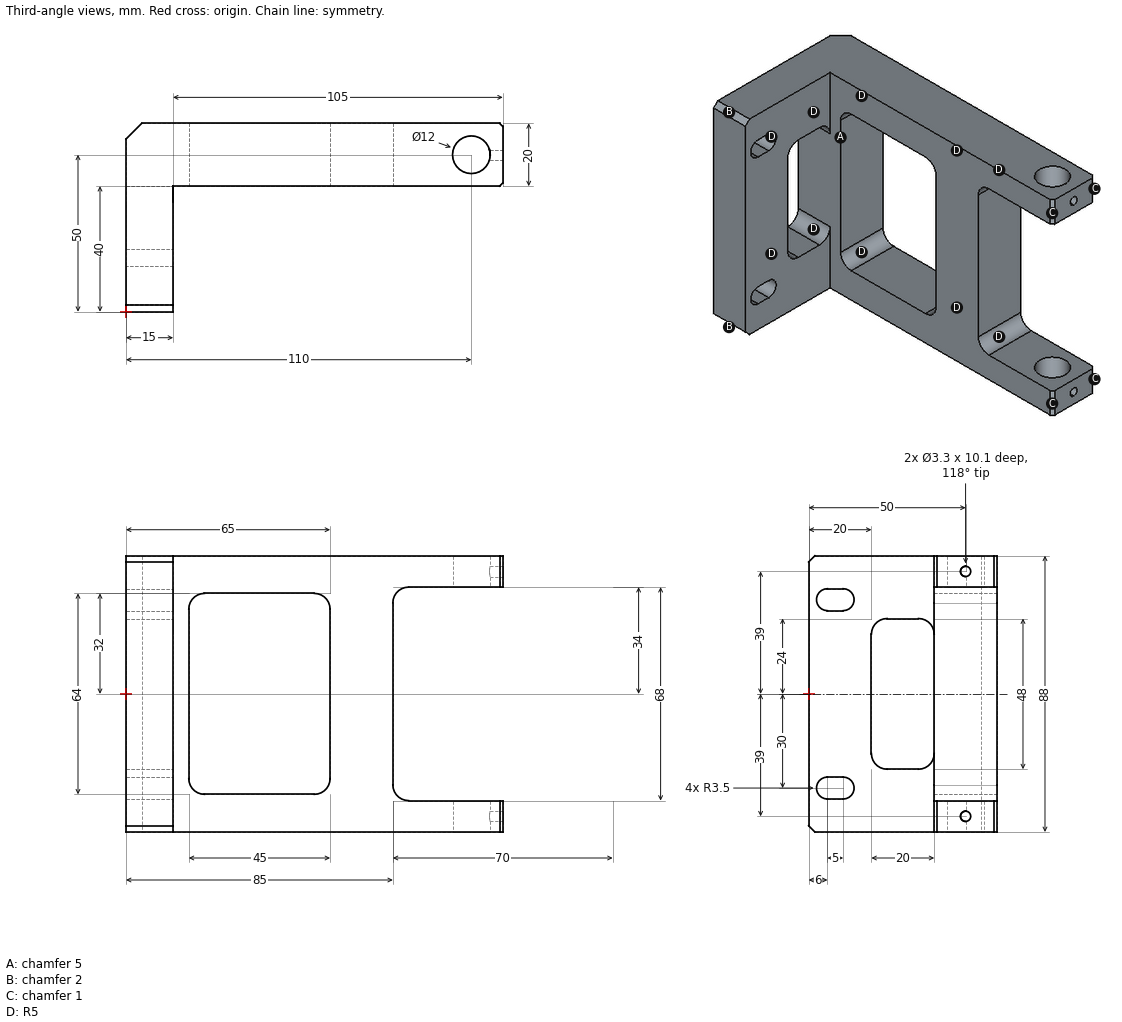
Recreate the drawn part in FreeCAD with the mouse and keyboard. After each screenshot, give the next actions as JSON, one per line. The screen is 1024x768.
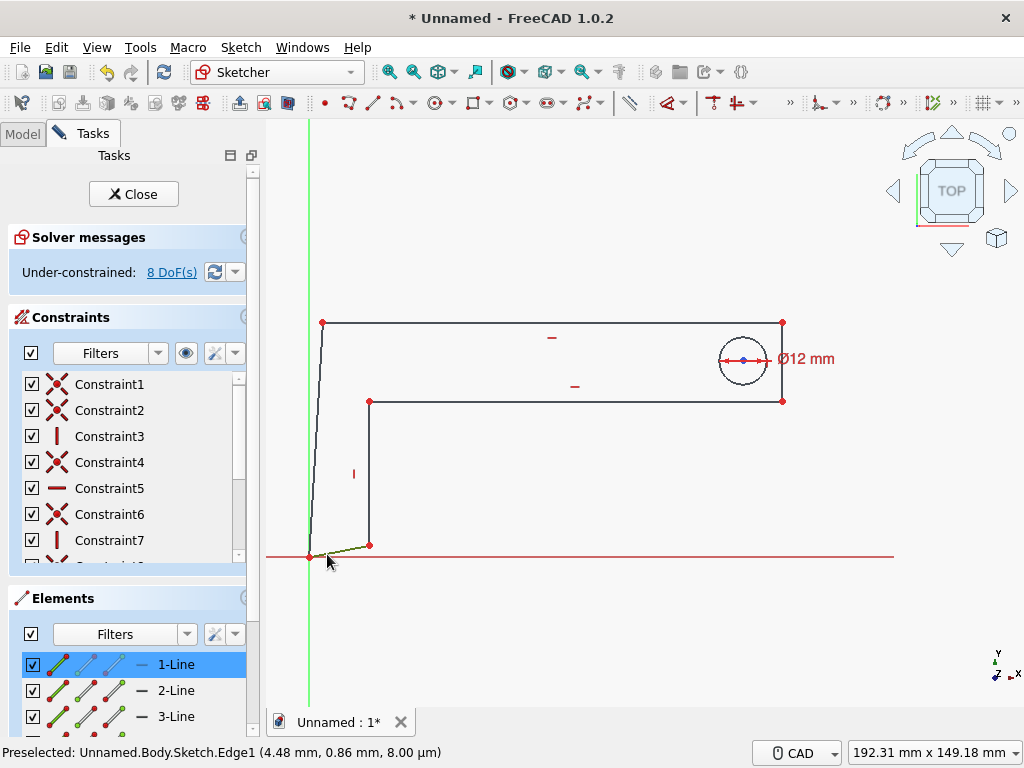
{"action": "left_click", "coordinate": [756, 104]}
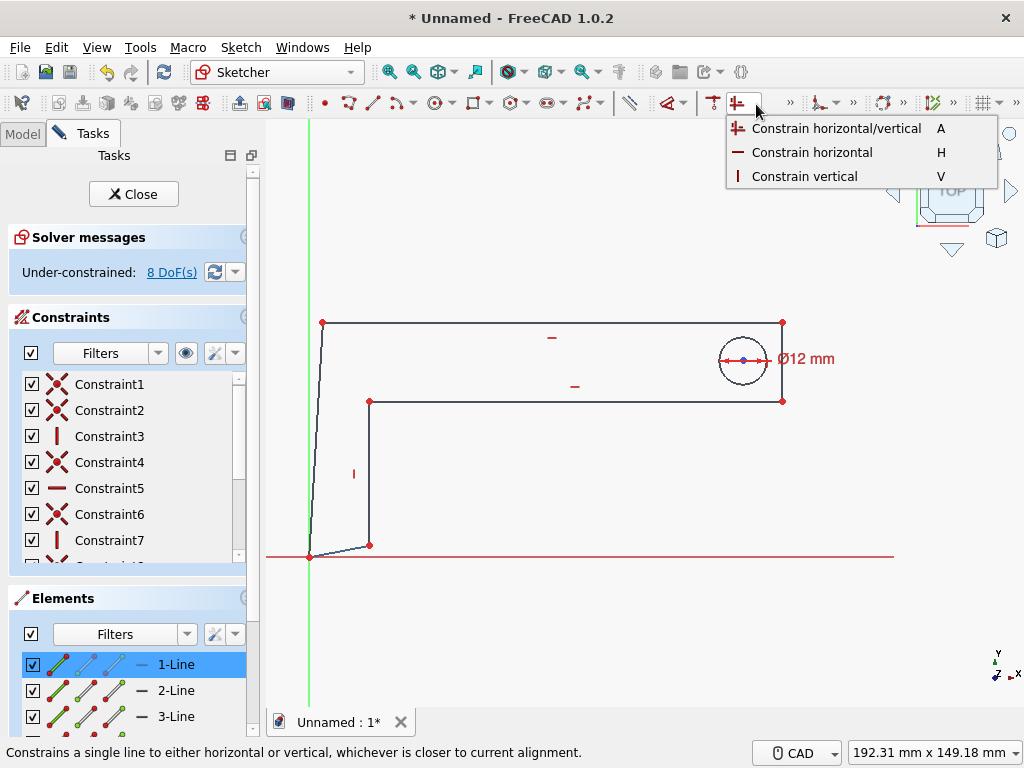
{"action": "left_click", "coordinate": [862, 152]}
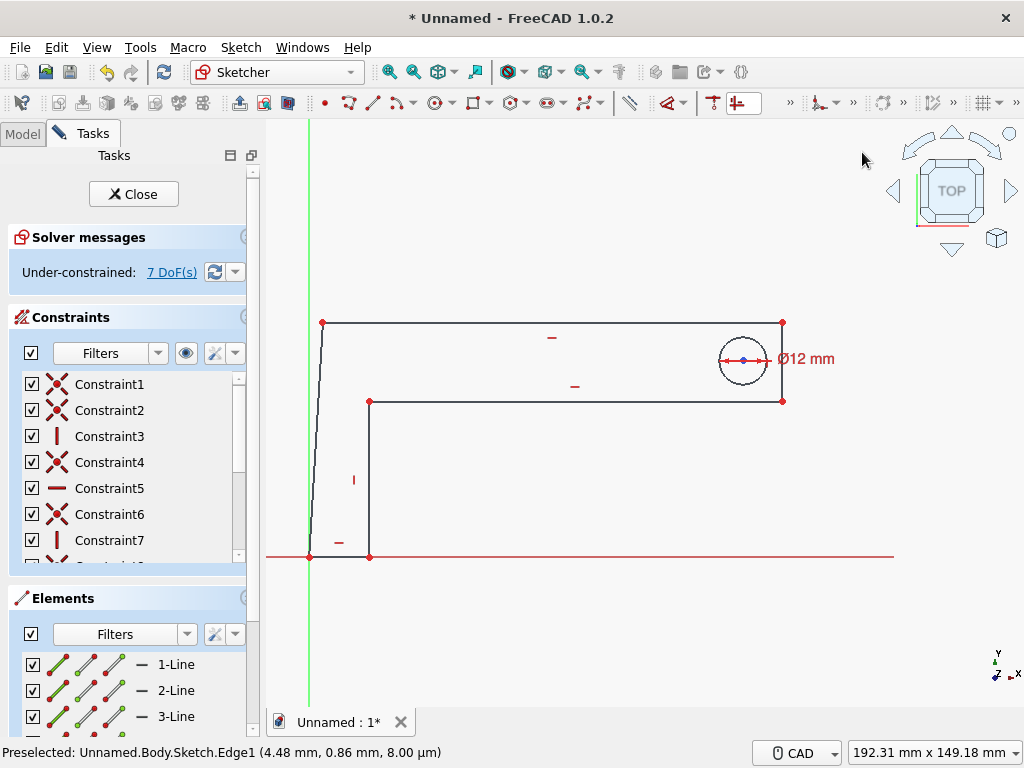
{"action": "scroll", "coordinate": [319, 393], "scroll_direction": "up", "scroll_amount": 2}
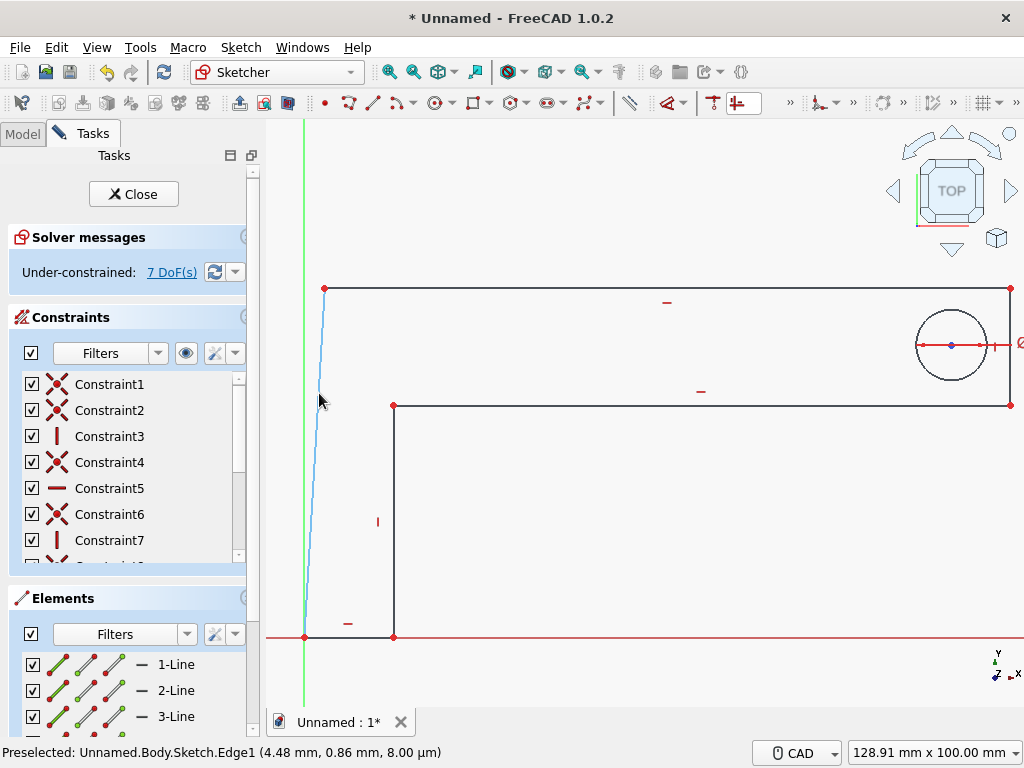
{"action": "left_click", "coordinate": [319, 393]}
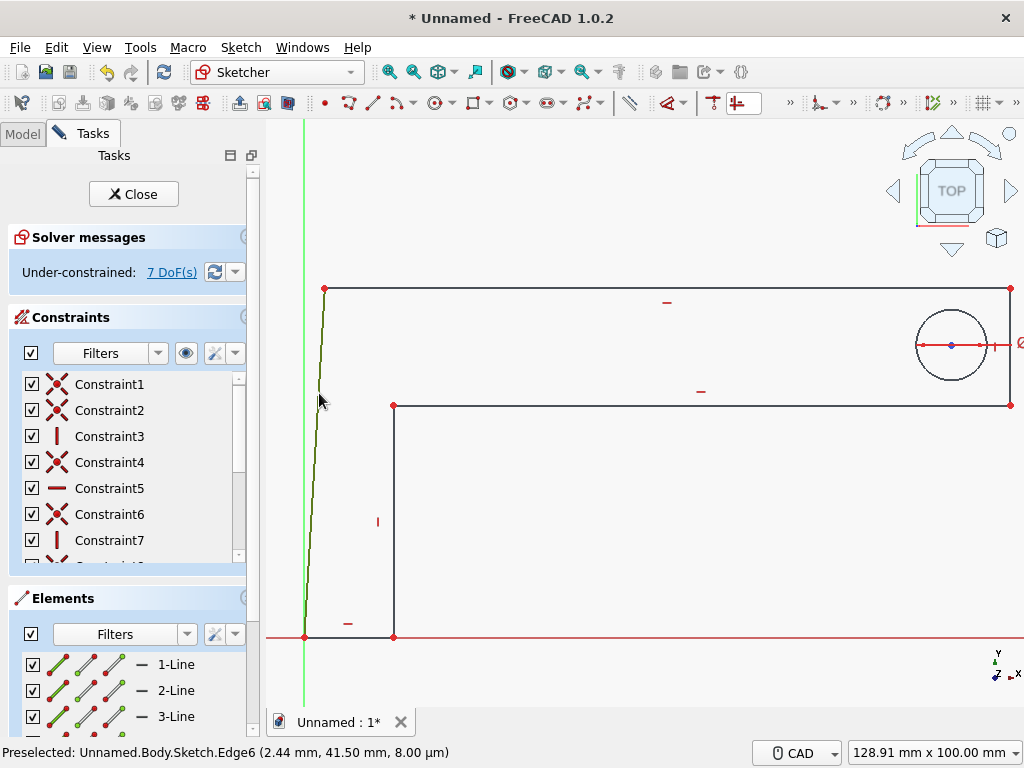
{"action": "key", "text": "v"}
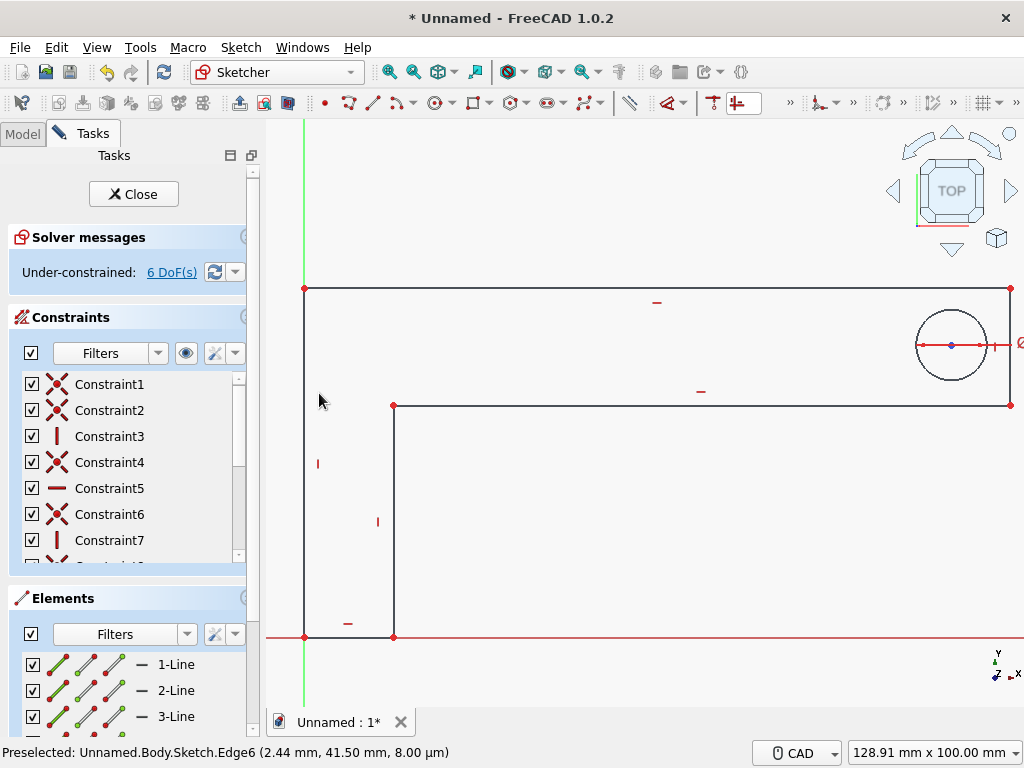
{"action": "left_click", "coordinate": [331, 638]}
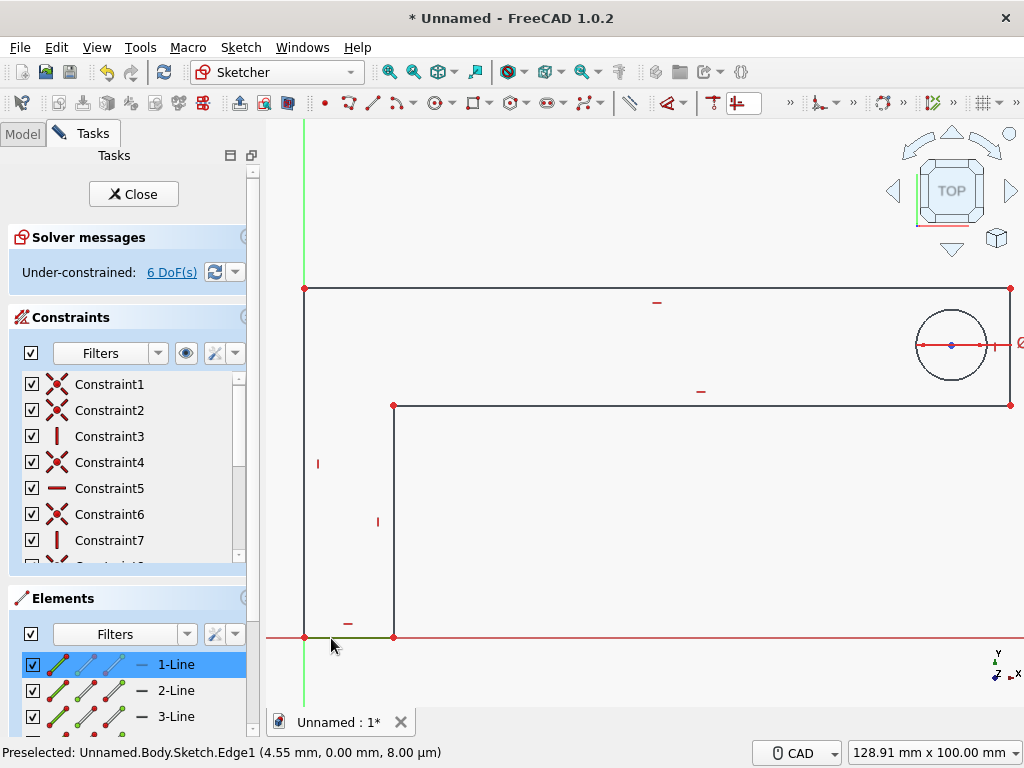
{"action": "key", "text": "l"}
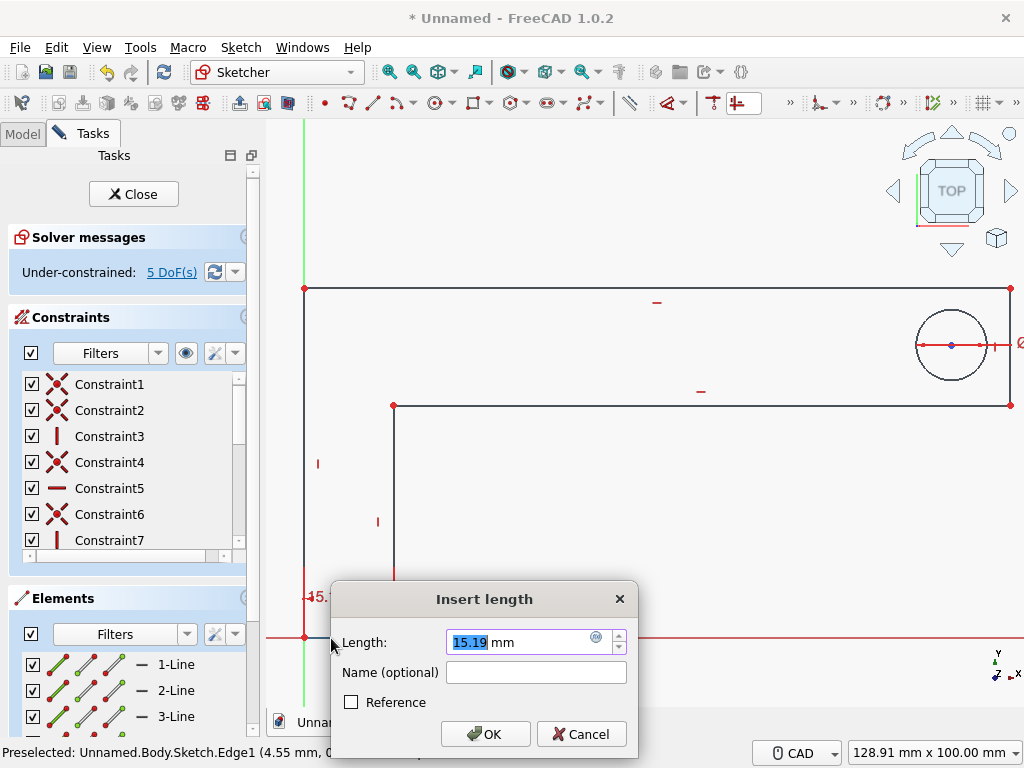
{"action": "type", "text": "15"}
{"action": "key", "text": "Return"}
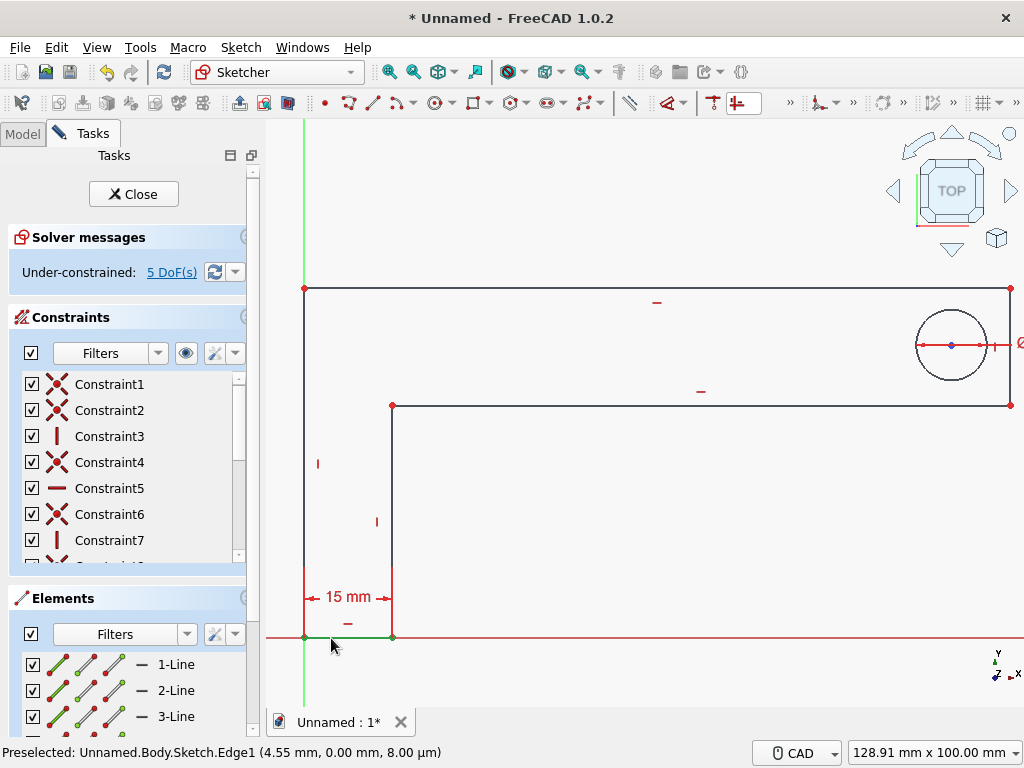
{"action": "left_click", "coordinate": [392, 568]}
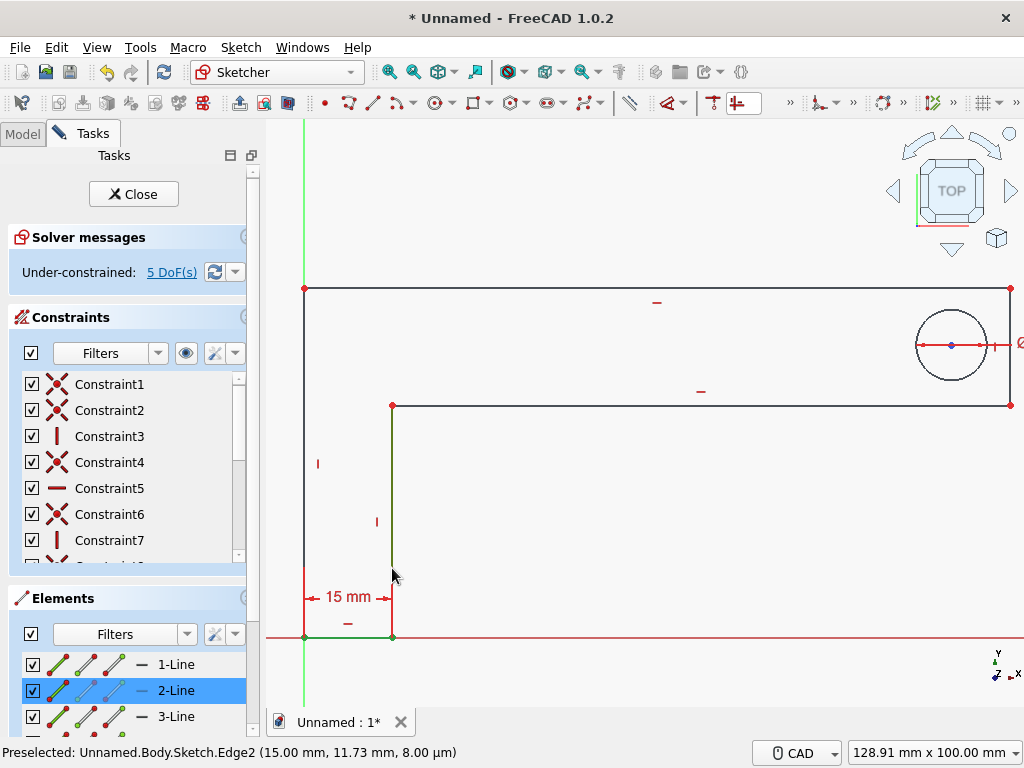
{"action": "key", "text": "i"}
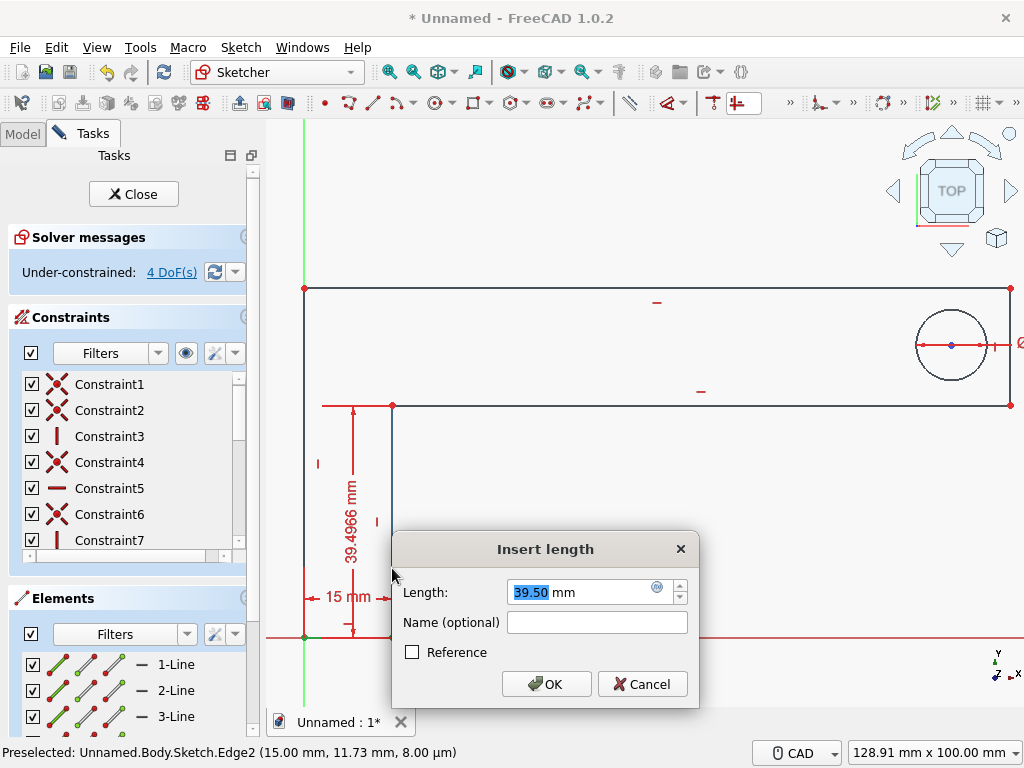
{"action": "type", "text": "40"}
{"action": "key", "text": "Return"}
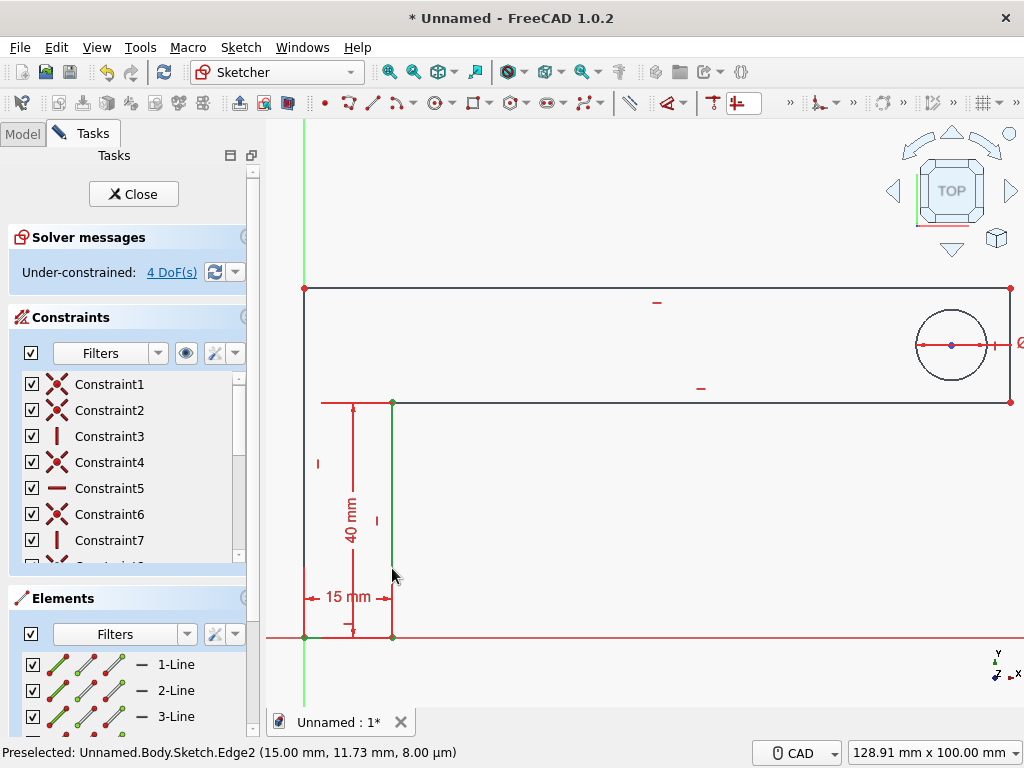
{"action": "scroll", "coordinate": [478, 354], "scroll_direction": "down", "scroll_amount": 3}